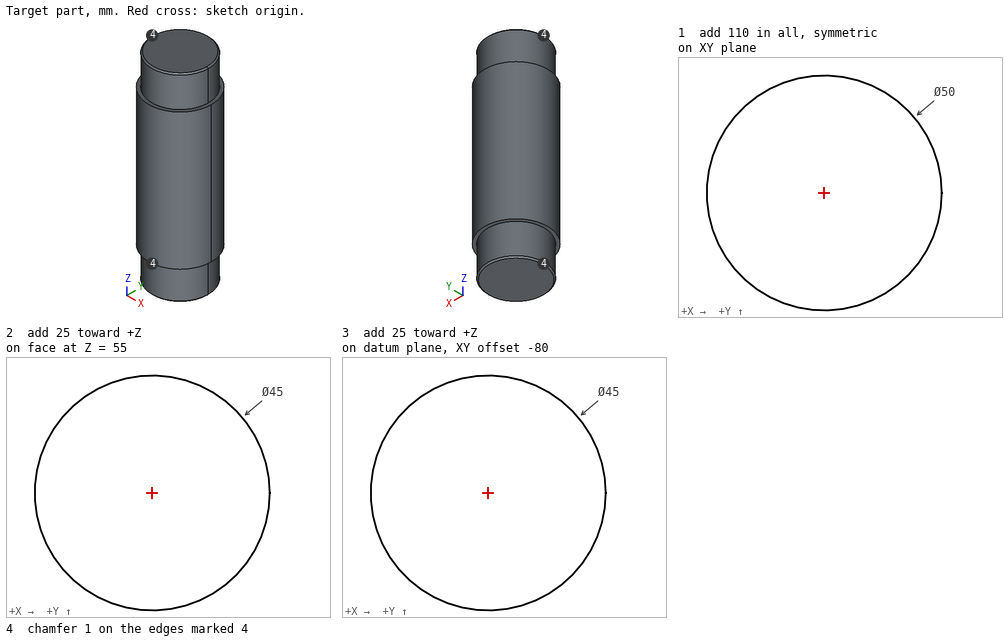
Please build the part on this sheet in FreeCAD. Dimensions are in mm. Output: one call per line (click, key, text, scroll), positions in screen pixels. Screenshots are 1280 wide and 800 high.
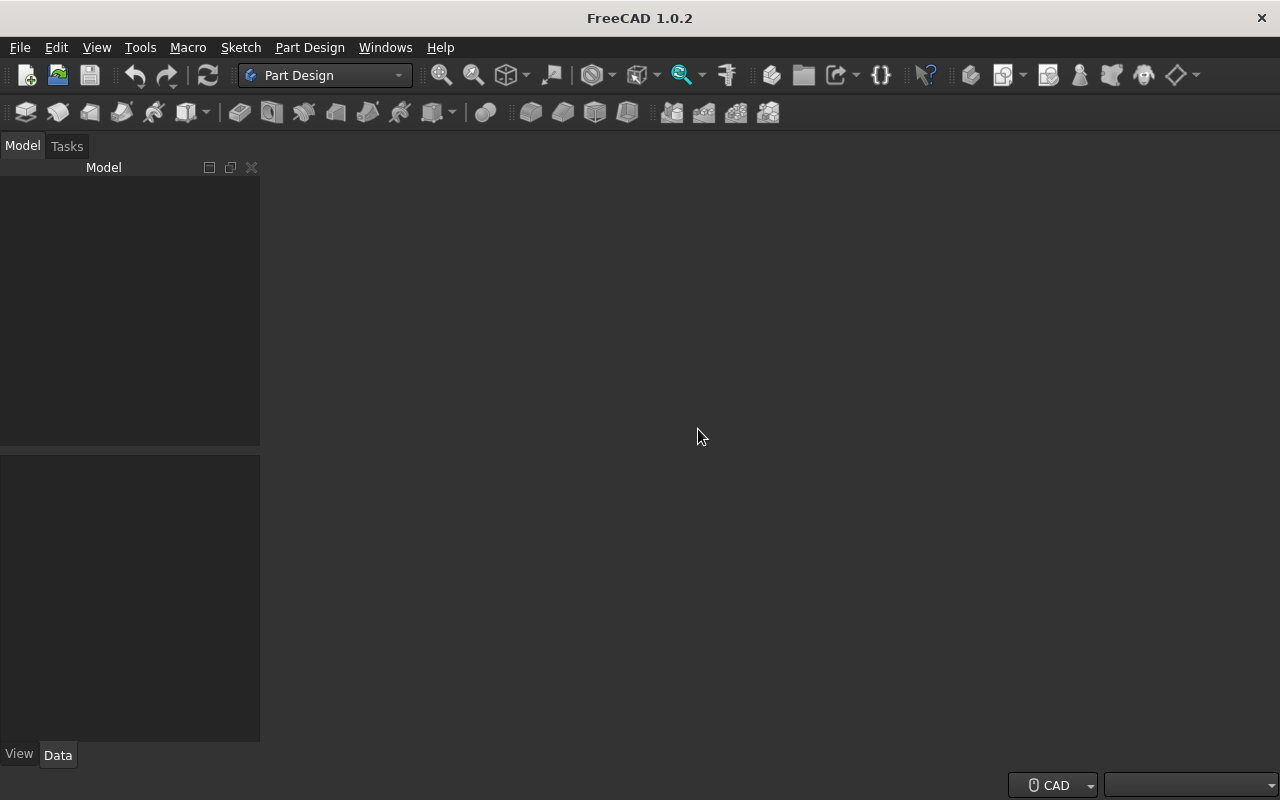
key(ctrl+n)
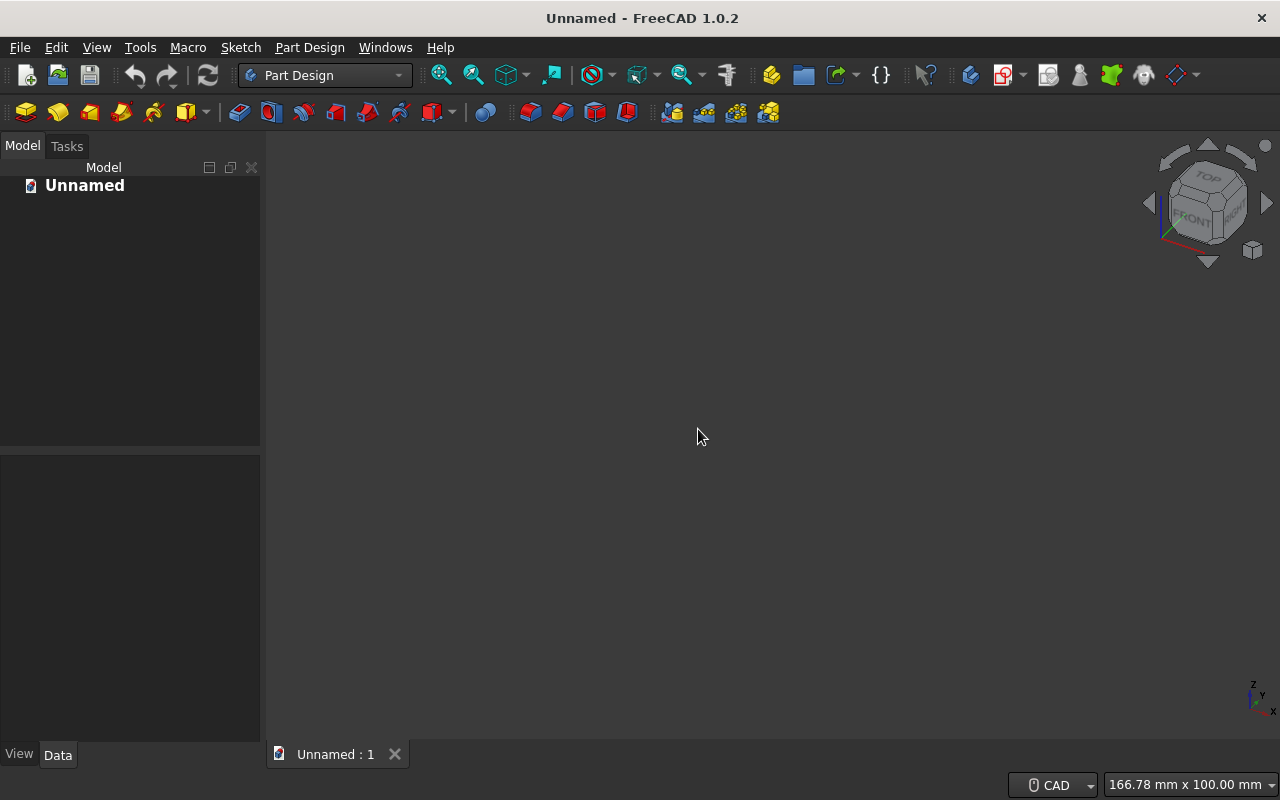
click(1004, 76)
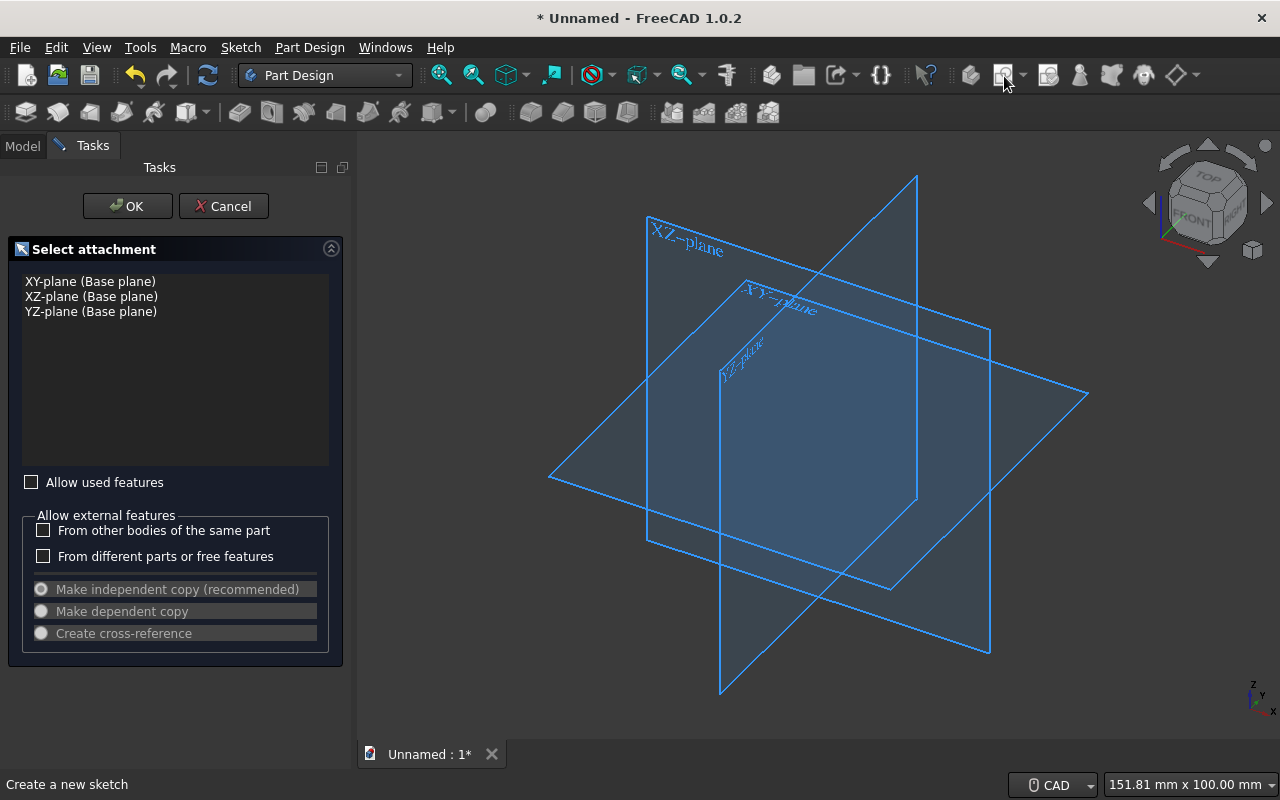
click(82, 282)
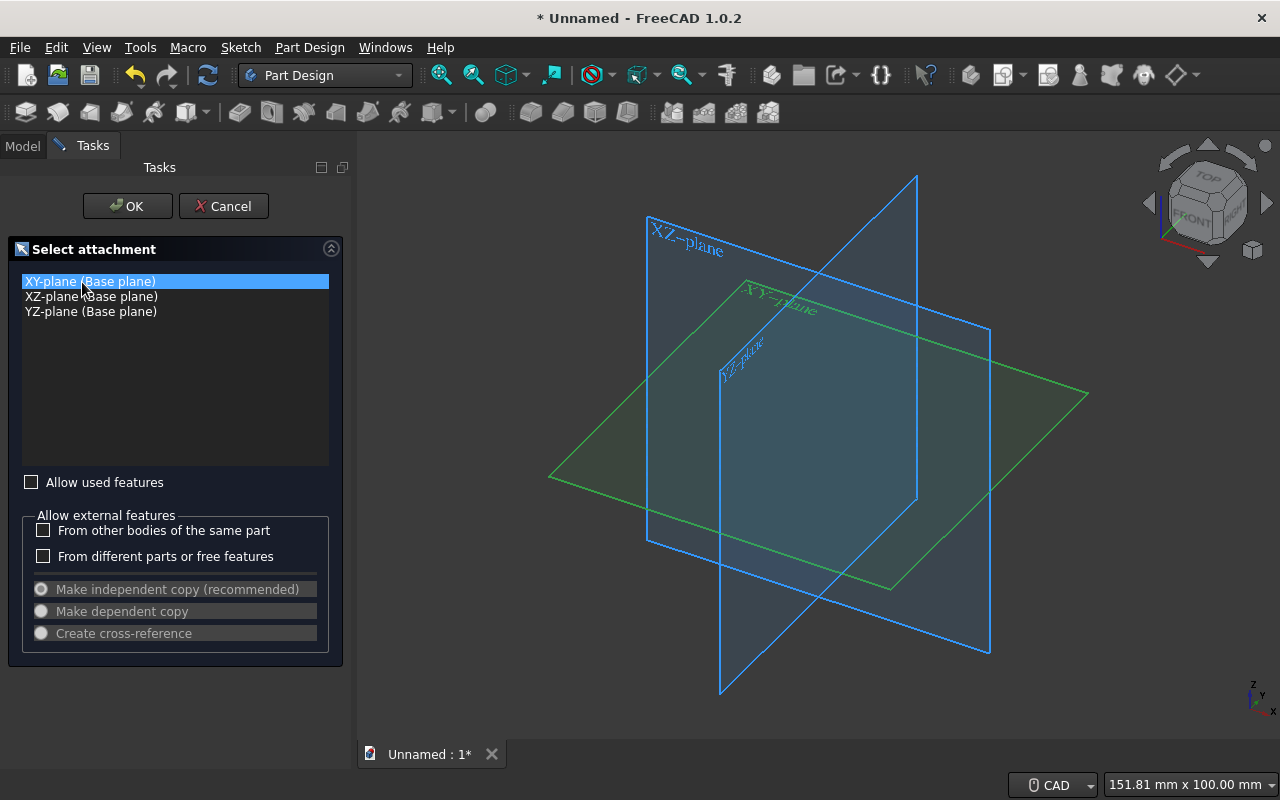
click(128, 206)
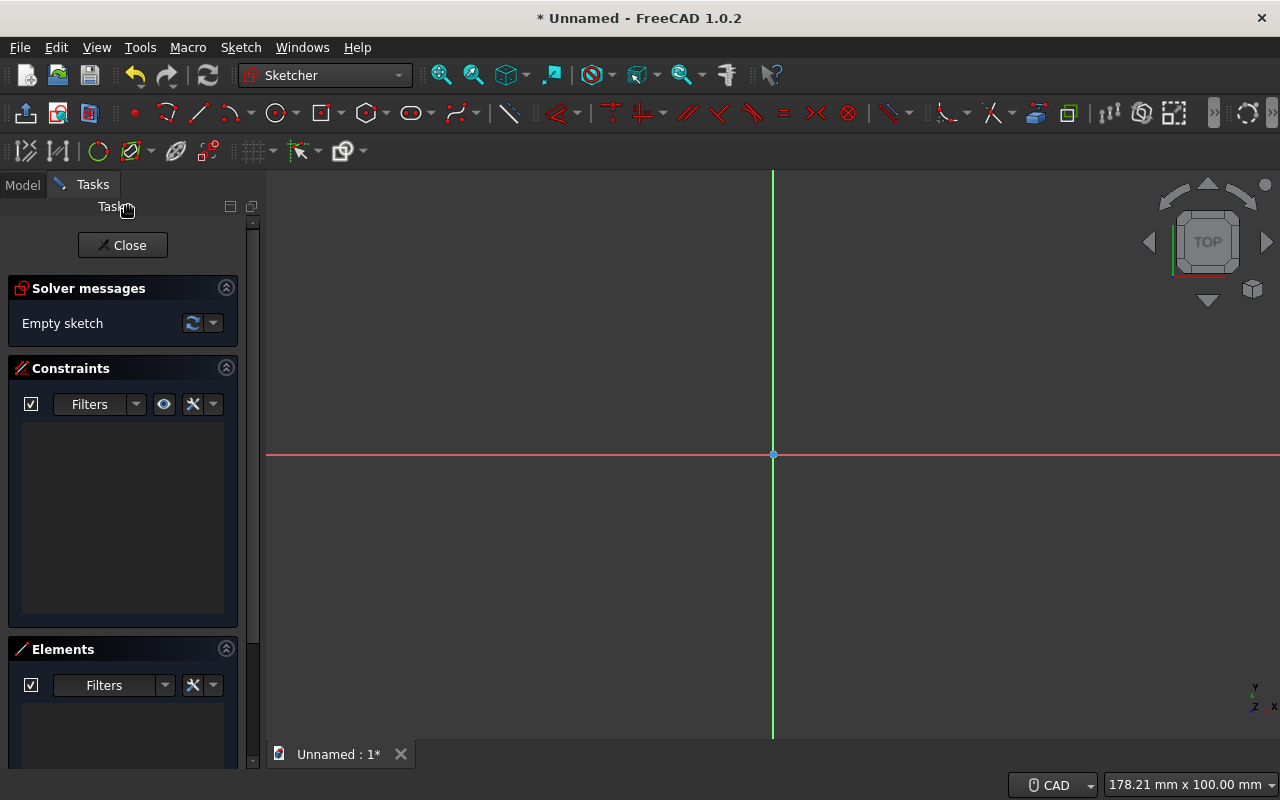
key(g)
key(c)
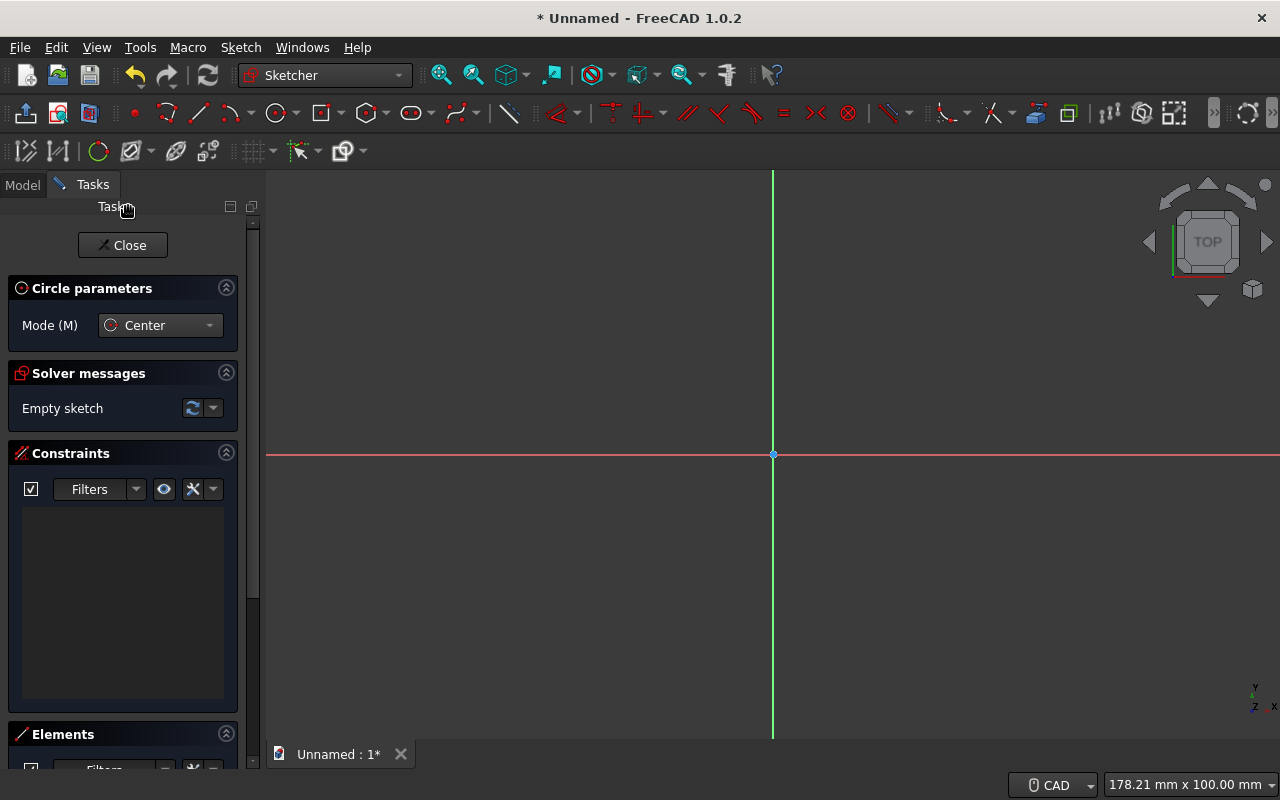
click(773, 454)
move(874, 354)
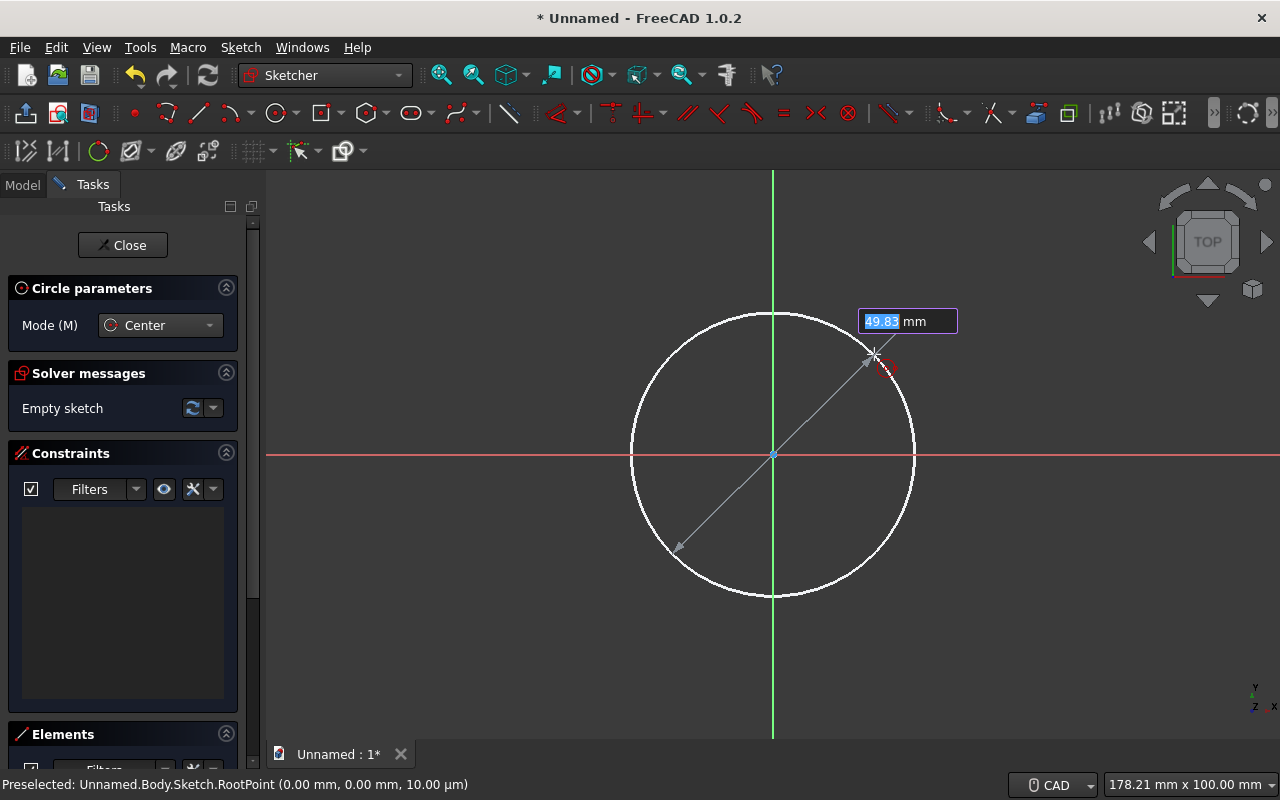
text(50)
key(Return)
key(Escape)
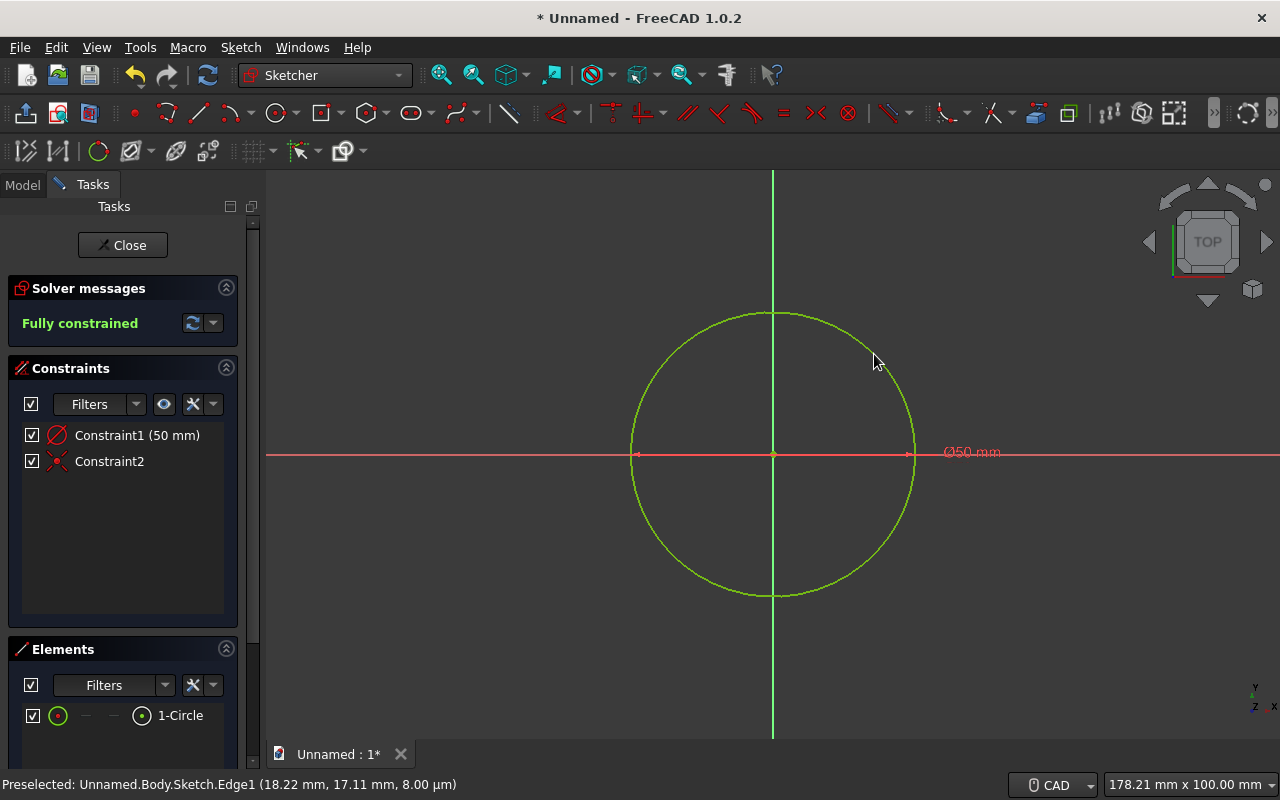
click(123, 245)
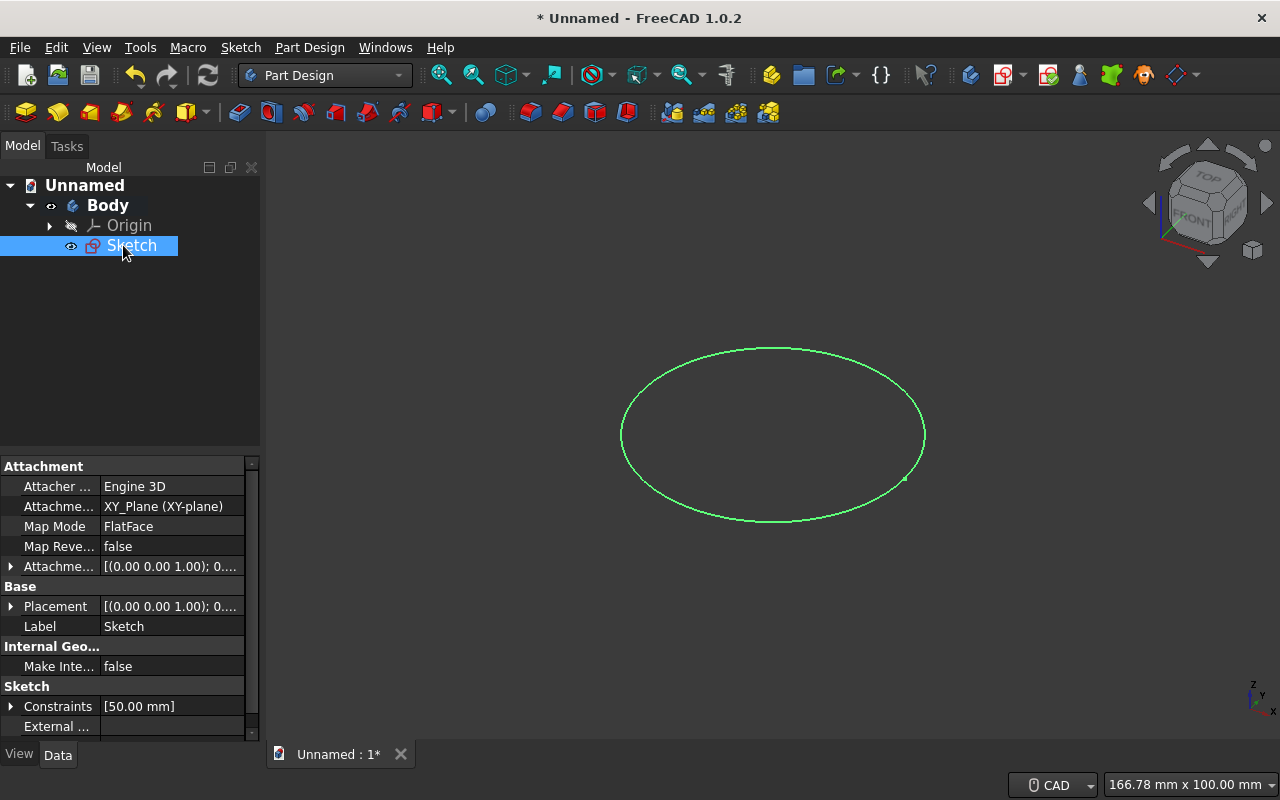
click(26, 112)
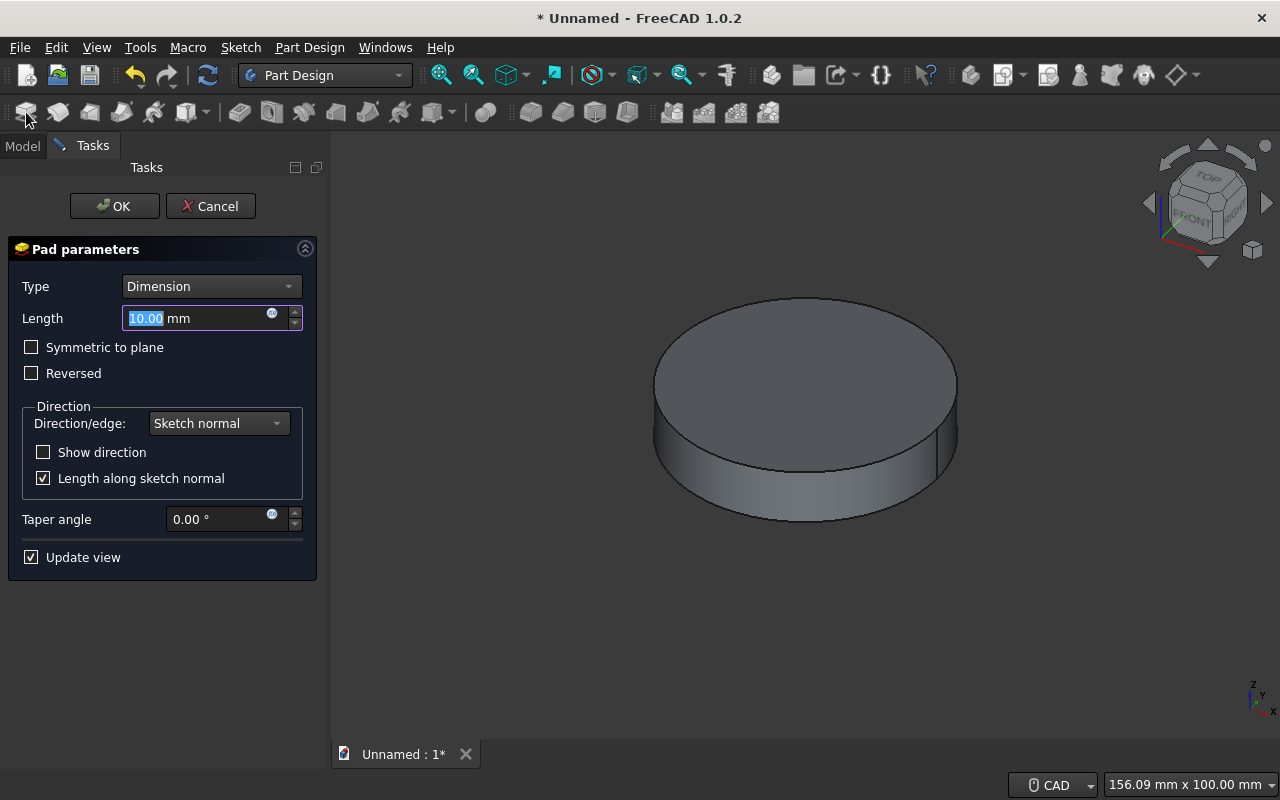
text(110)
key(Tab)